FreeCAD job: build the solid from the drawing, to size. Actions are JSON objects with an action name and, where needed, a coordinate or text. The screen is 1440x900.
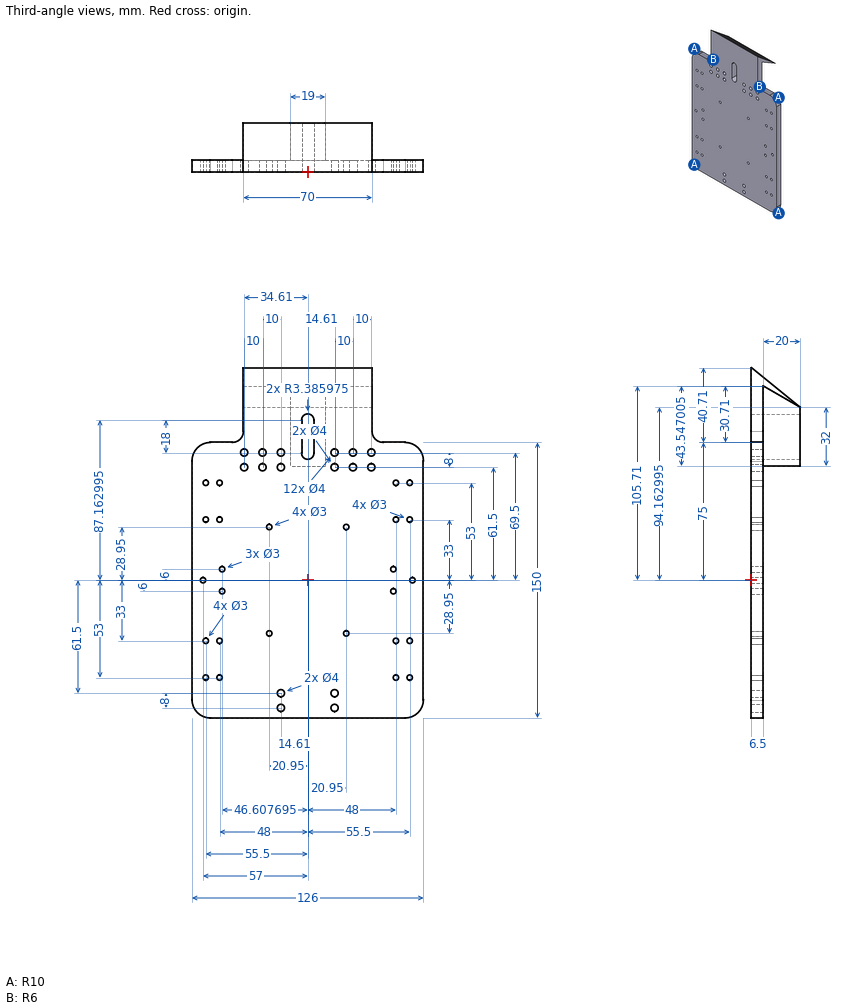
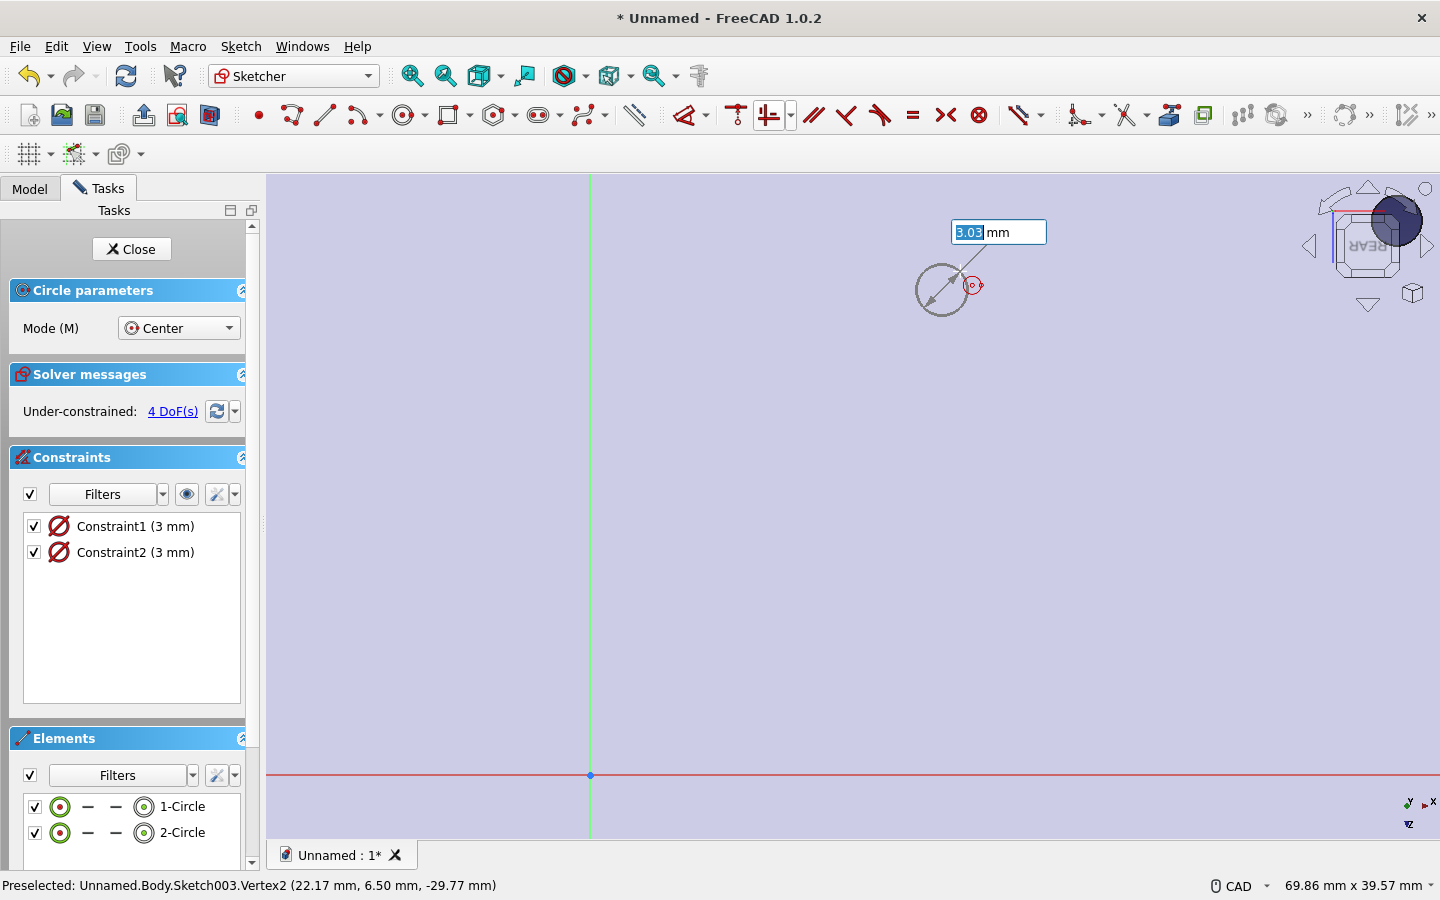
{"action": "type", "text": "3"}
{"action": "key", "text": "Return"}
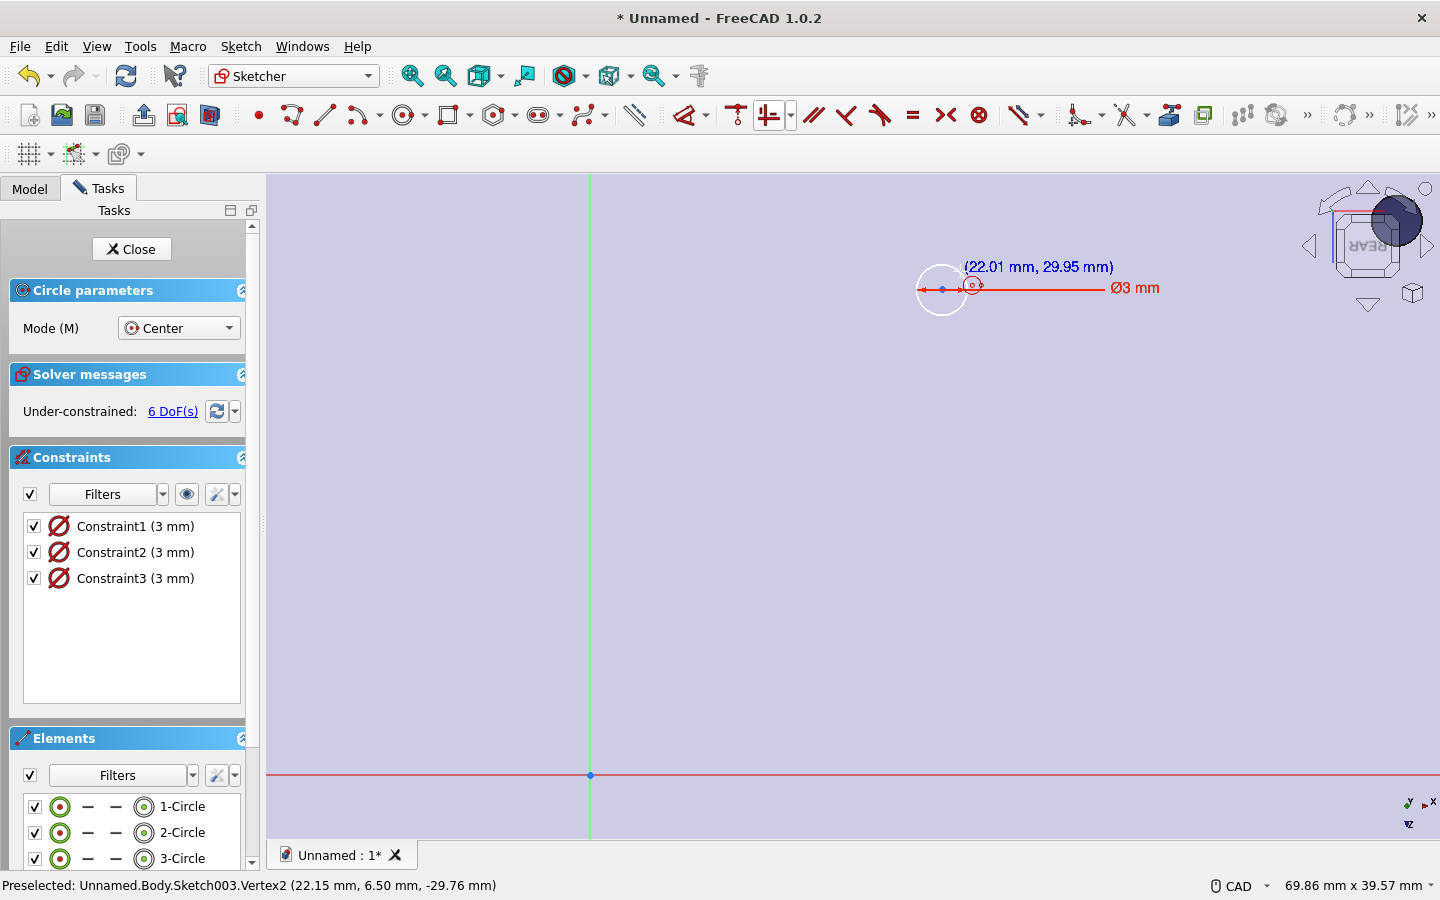
{"action": "scroll", "coordinate": [943, 287], "scroll_direction": "down", "scroll_amount": 4}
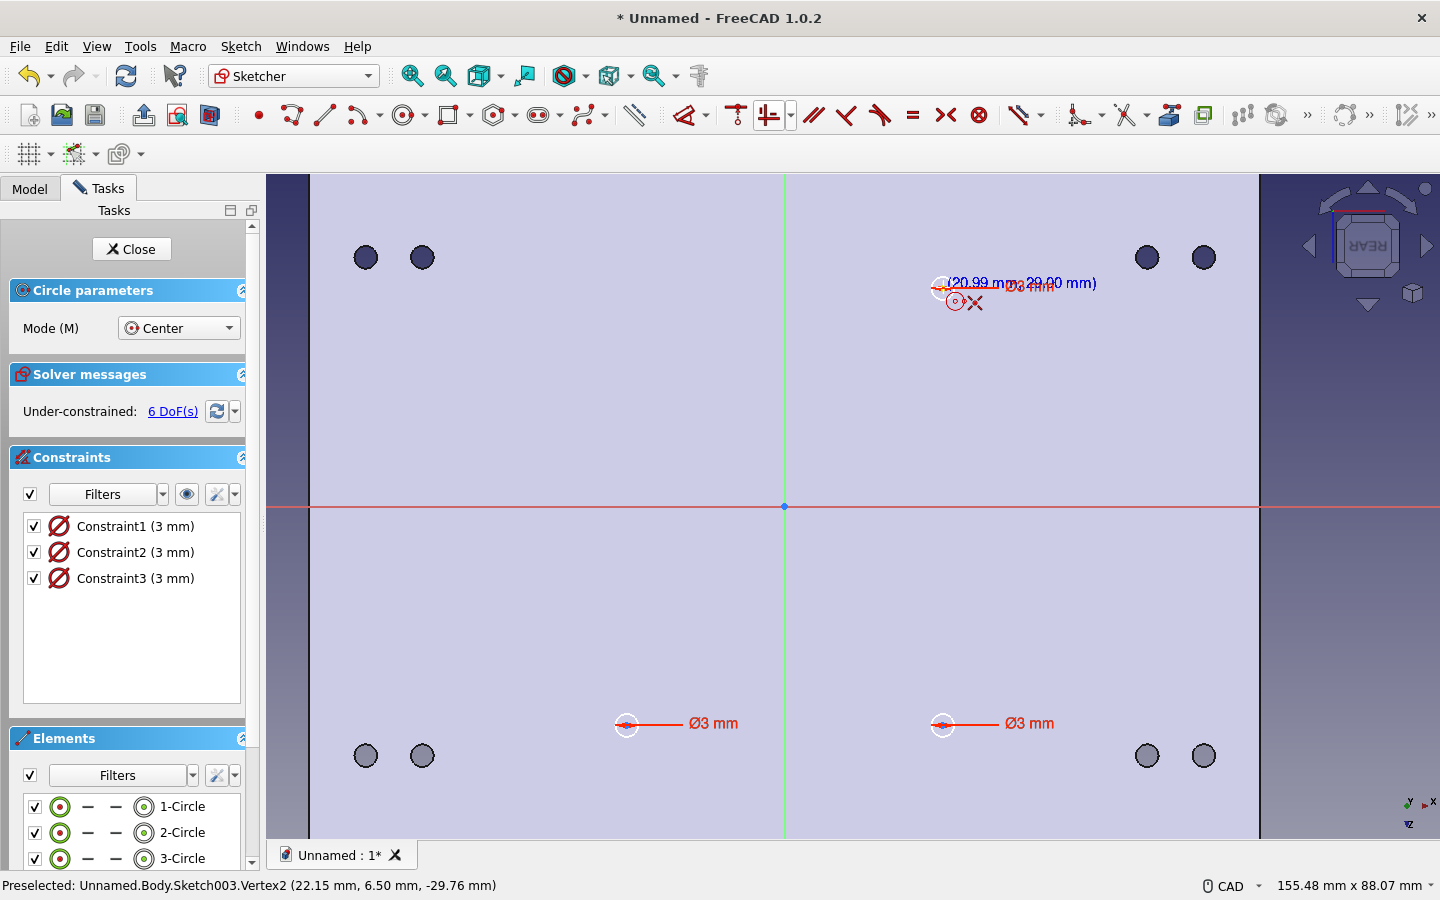
{"action": "scroll", "coordinate": [627, 288], "scroll_direction": "up", "scroll_amount": 4}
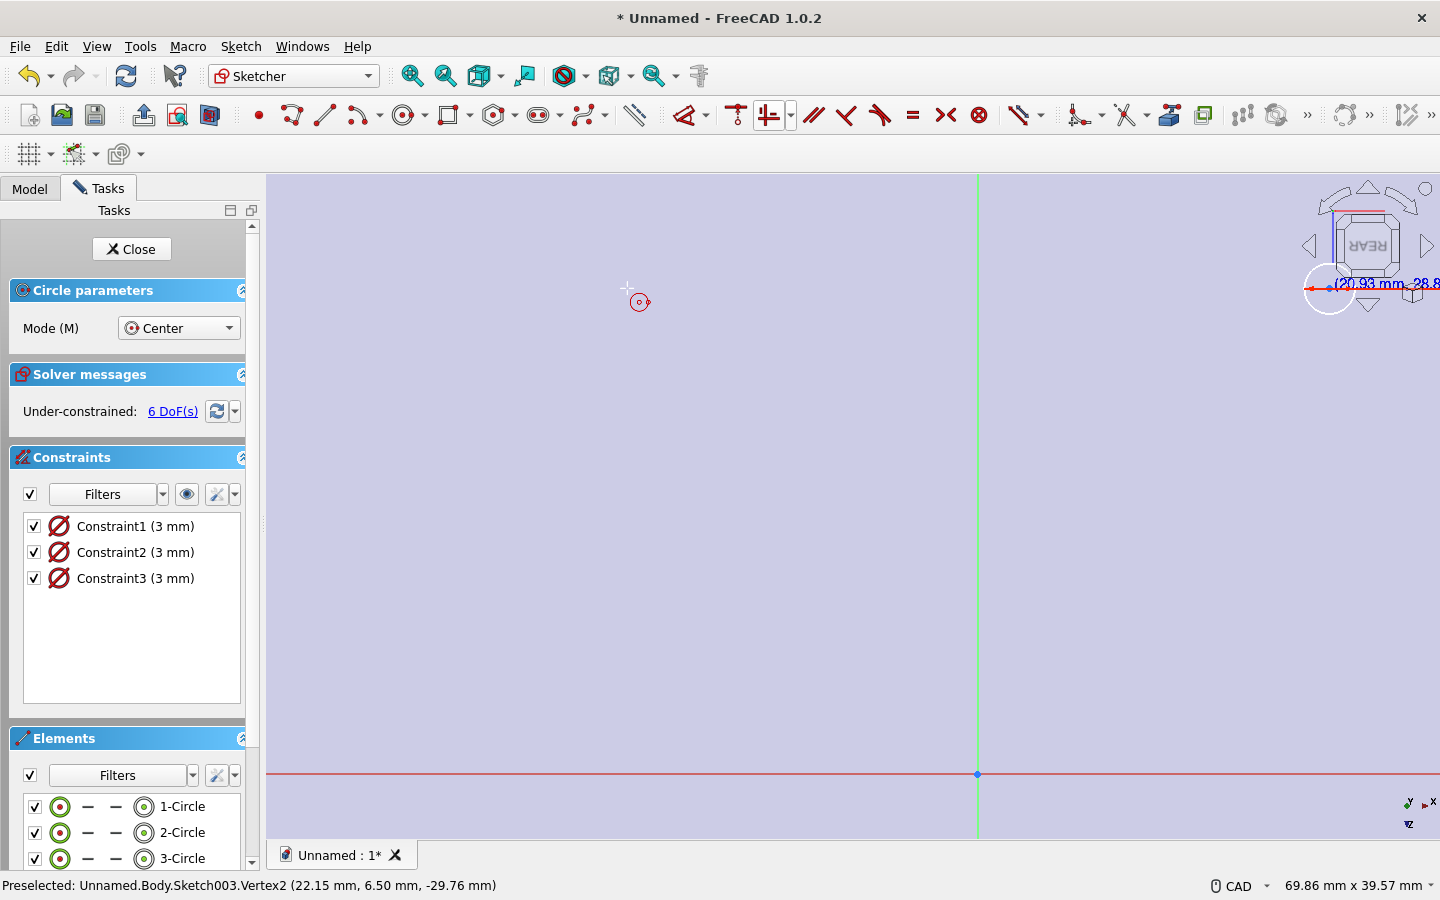
{"action": "left_click", "coordinate": [626, 288]}
{"action": "mouse_move", "coordinate": [644, 270]}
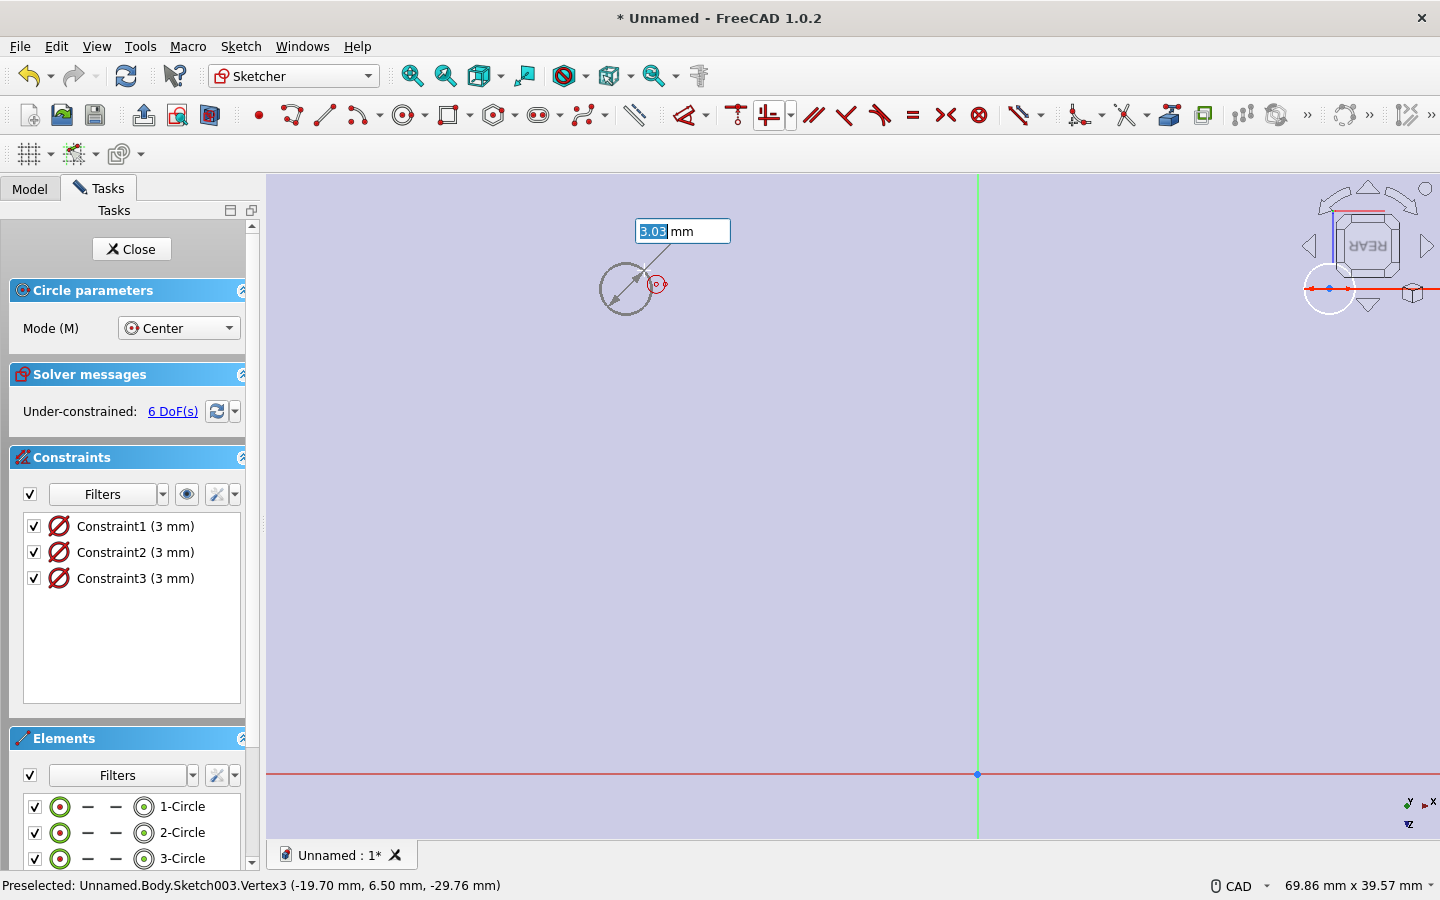
{"action": "type", "text": "3"}
{"action": "key", "text": "Return"}
{"action": "key", "text": "Escape"}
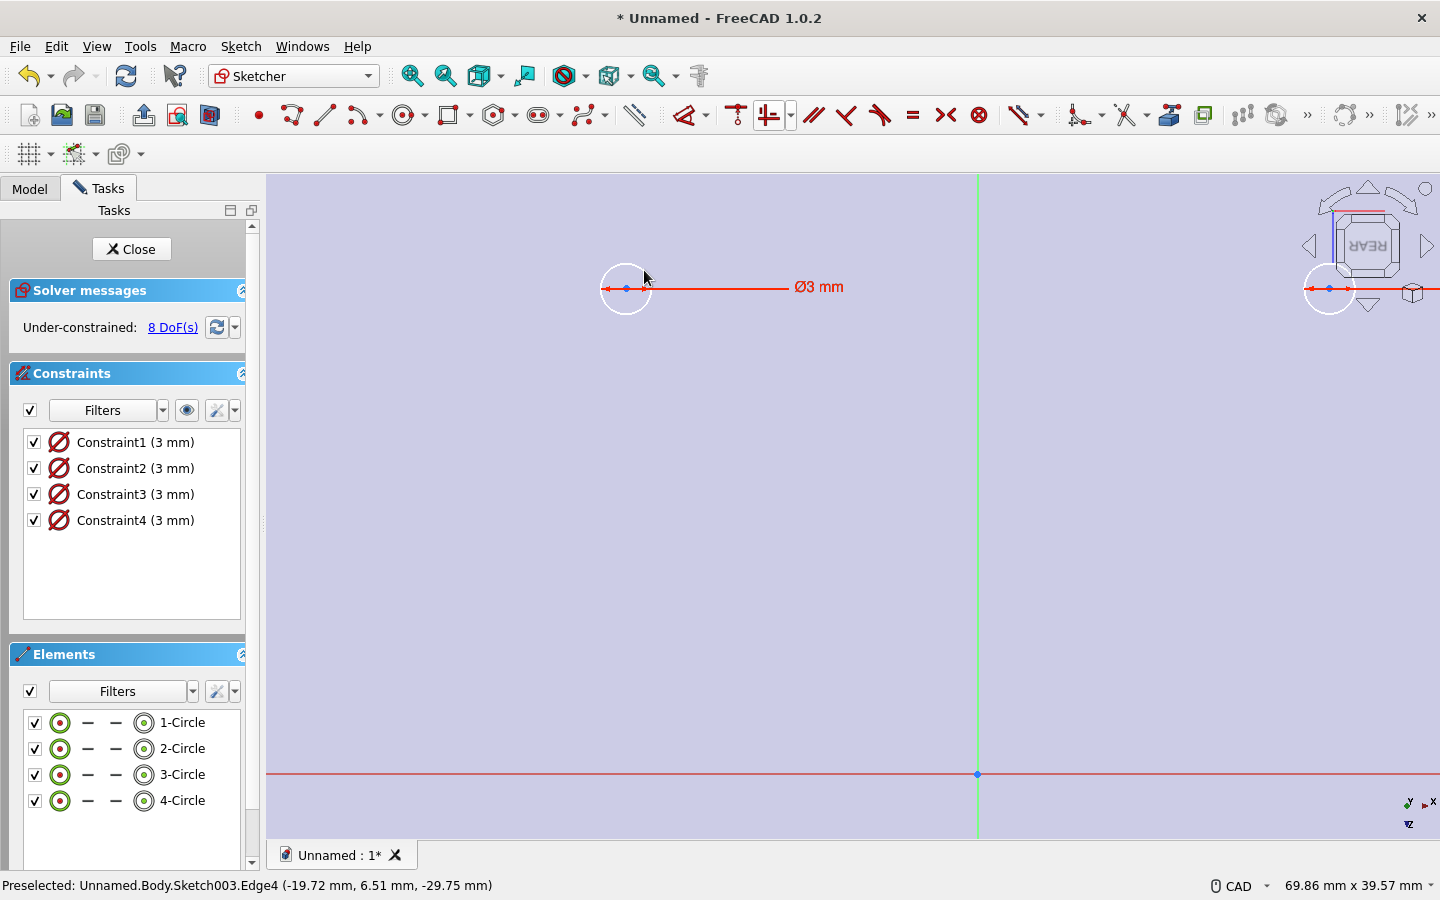
{"action": "scroll", "coordinate": [627, 288], "scroll_direction": "down", "scroll_amount": 4}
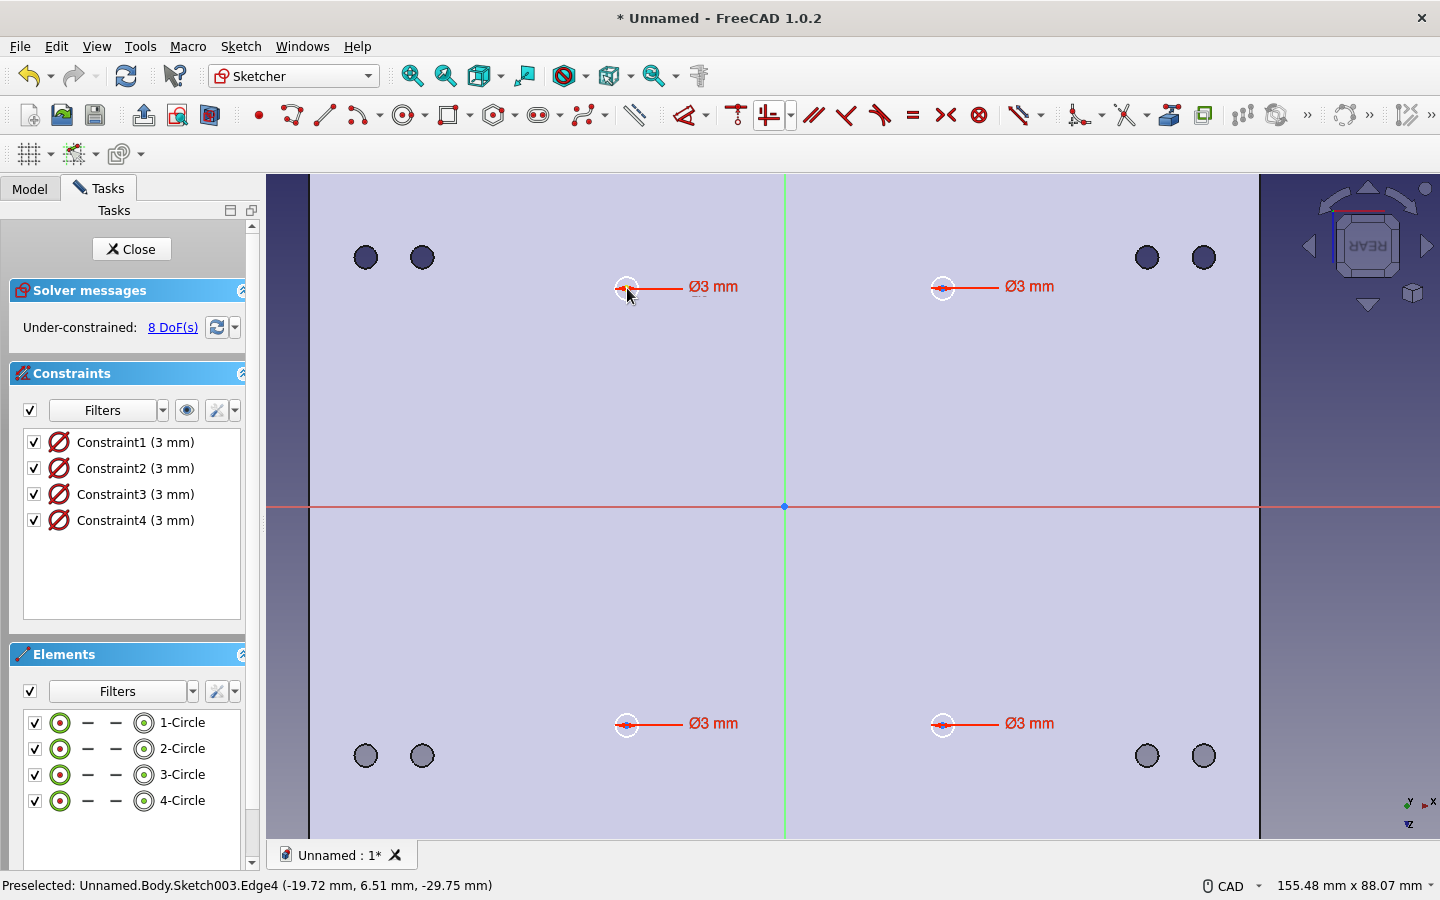
{"action": "left_click", "coordinate": [627, 725]}